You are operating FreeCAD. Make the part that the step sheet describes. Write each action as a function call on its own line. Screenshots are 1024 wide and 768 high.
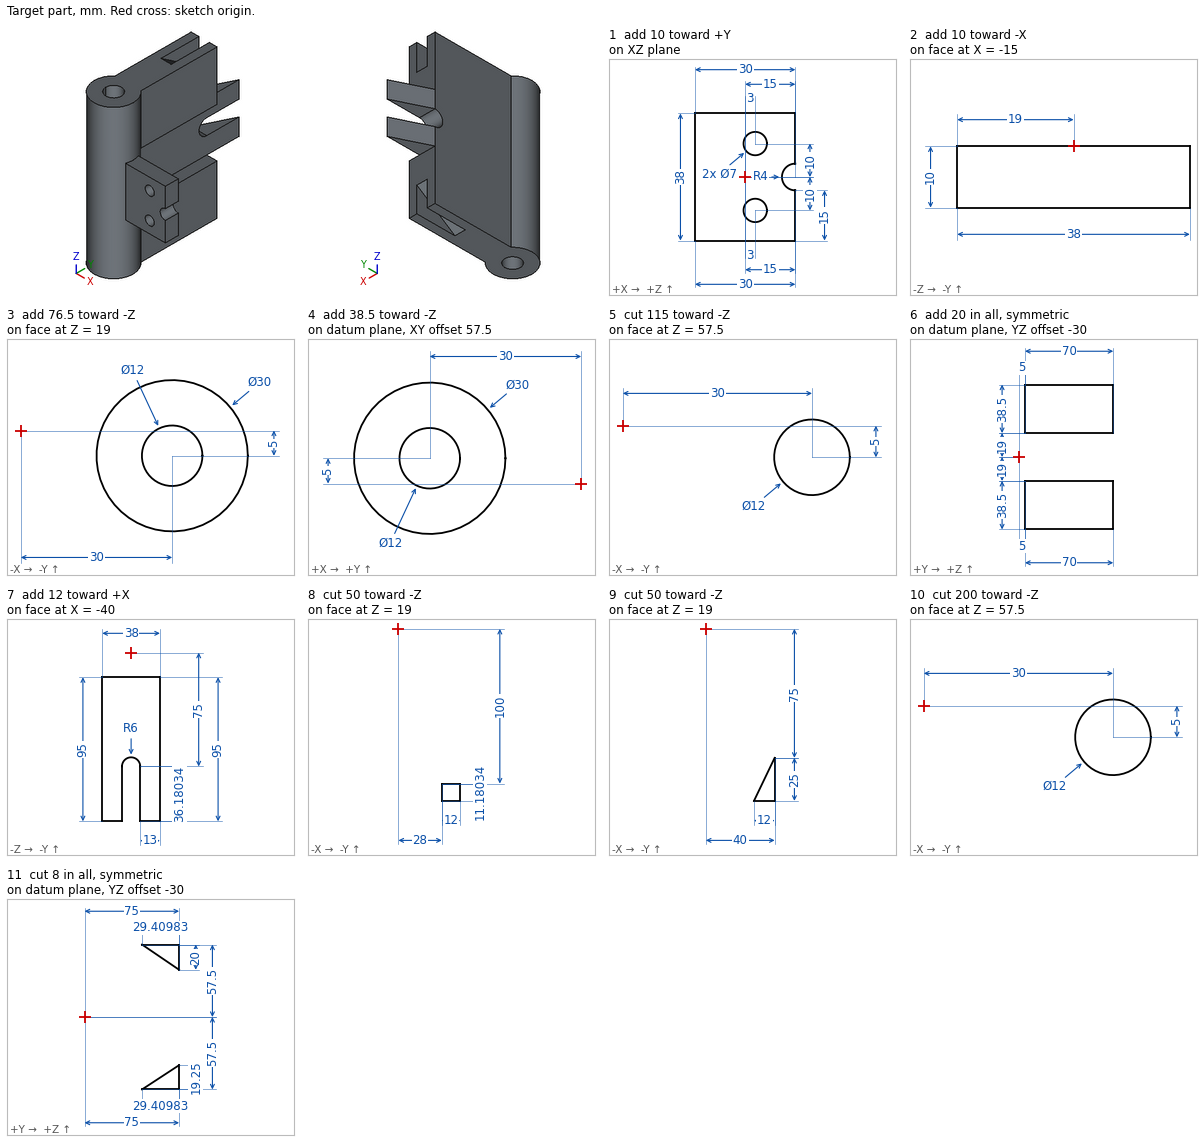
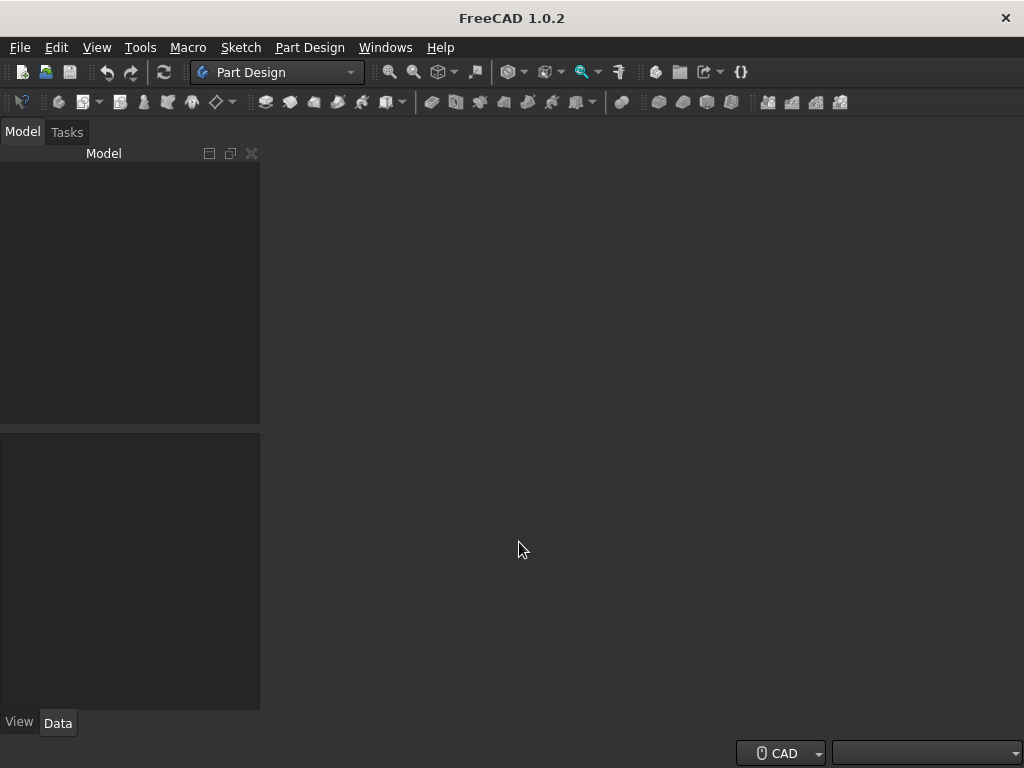
click(22, 72)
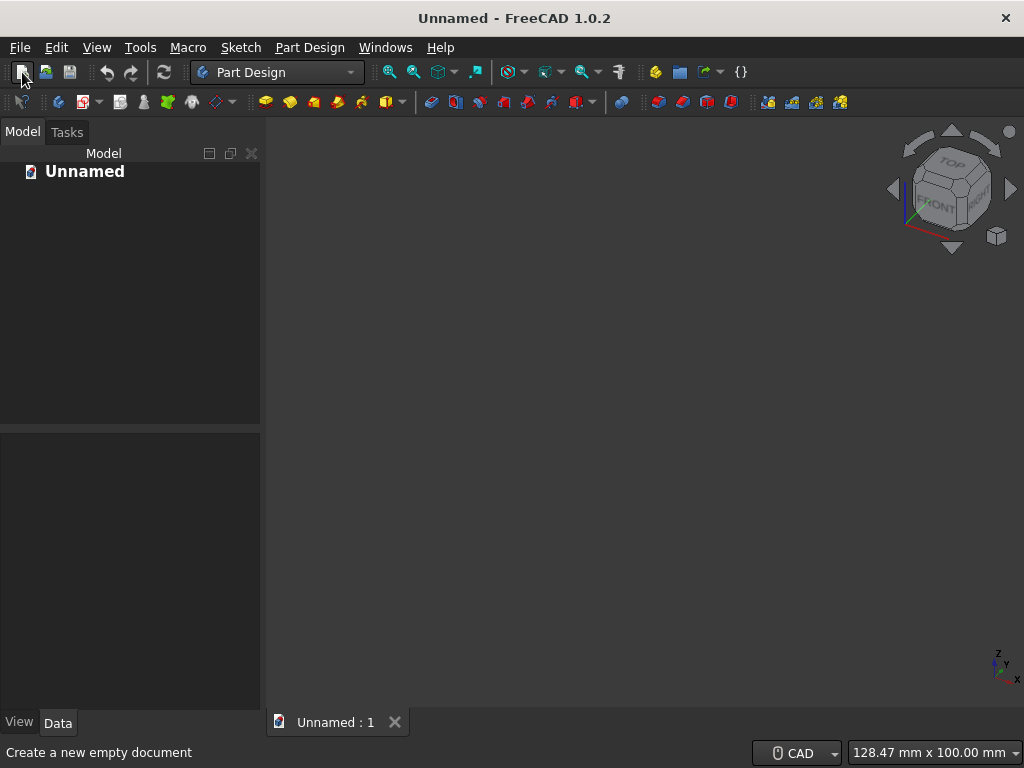
click(84, 102)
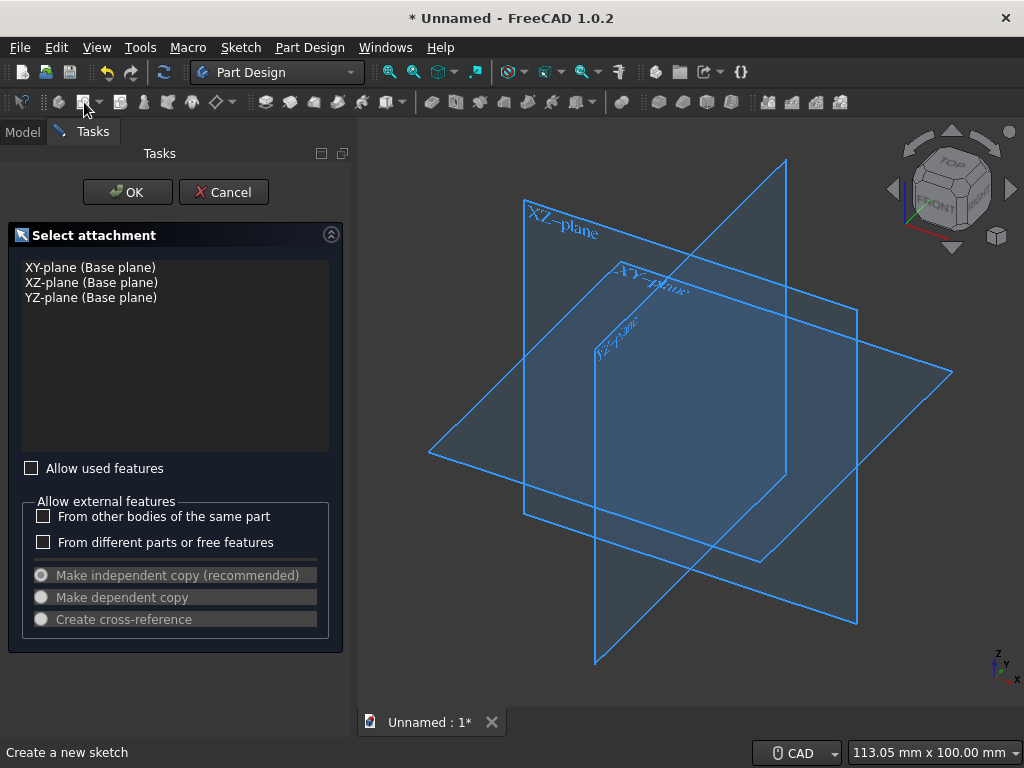
click(82, 282)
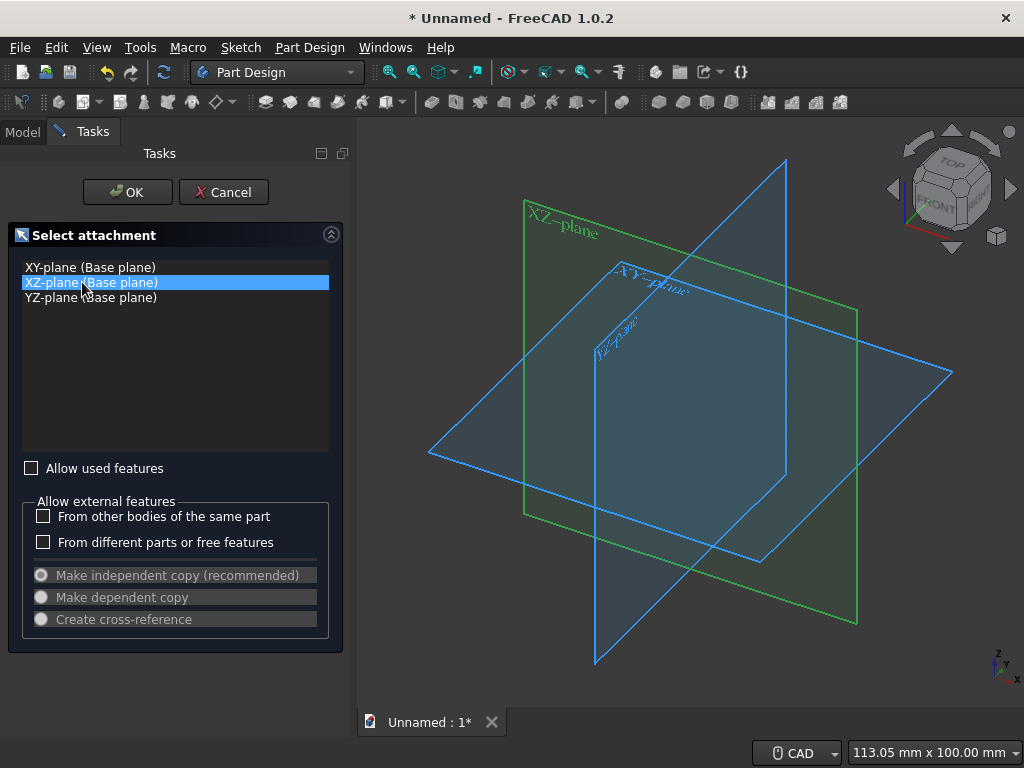
click(128, 192)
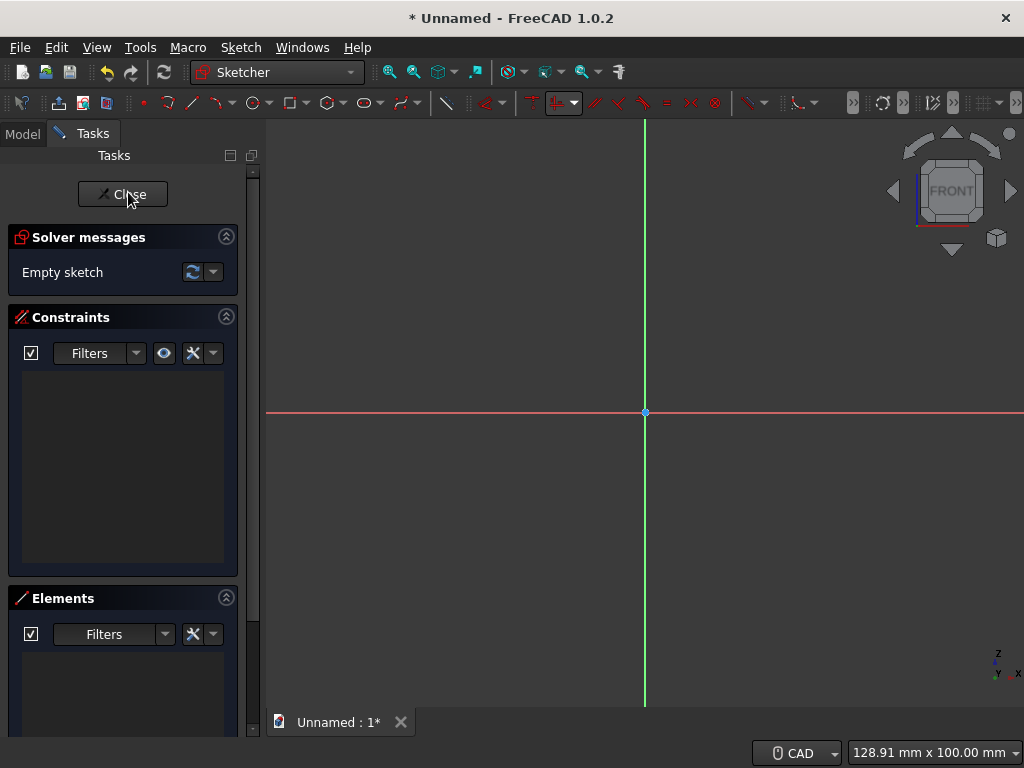
scroll(728, 413, up, 3)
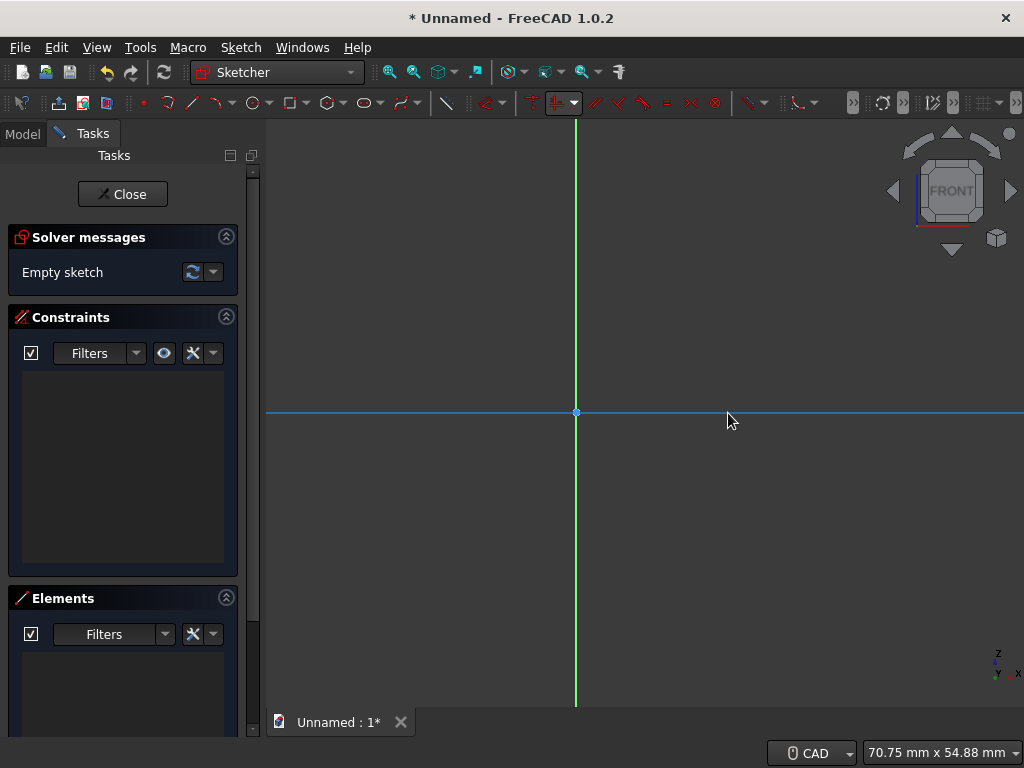
key(g)
key(m)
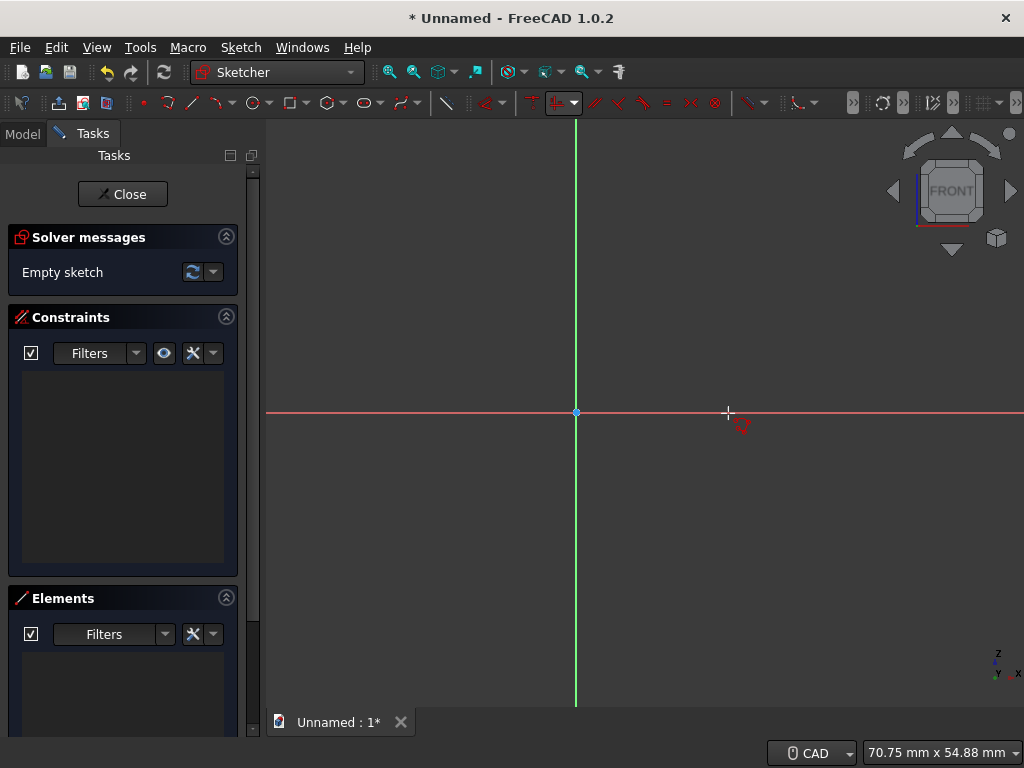
click(737, 455)
click(737, 616)
click(416, 616)
click(416, 209)
click(737, 209)
click(737, 370)
right_click(737, 370)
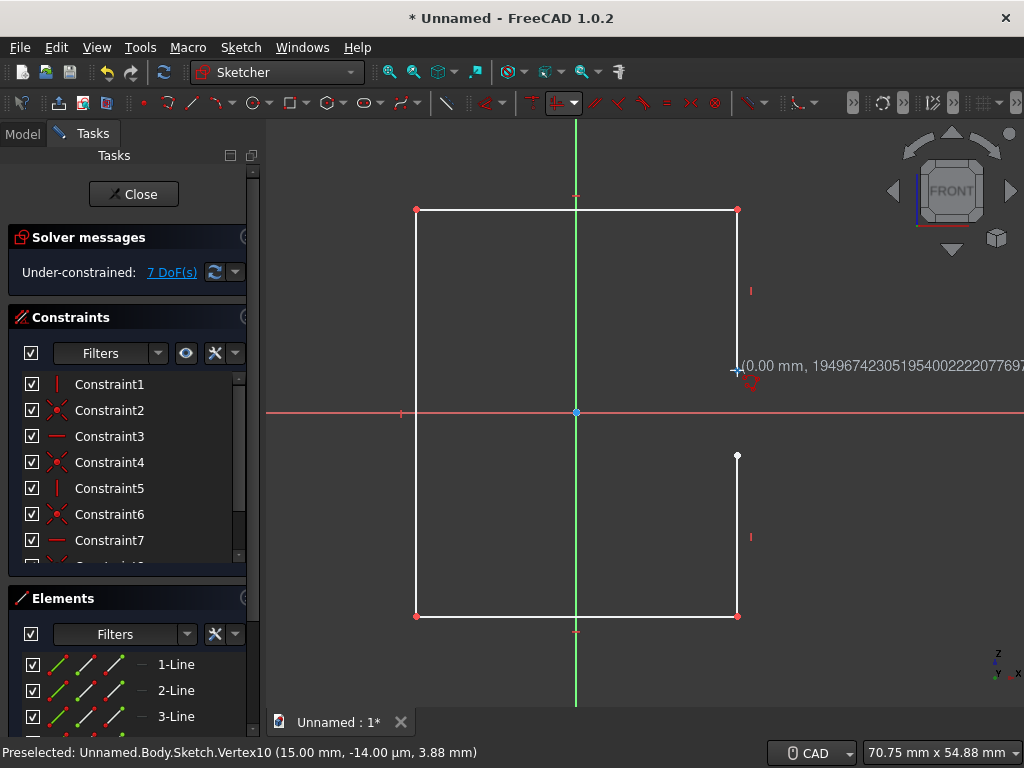
key(g)
key(3)
key(a)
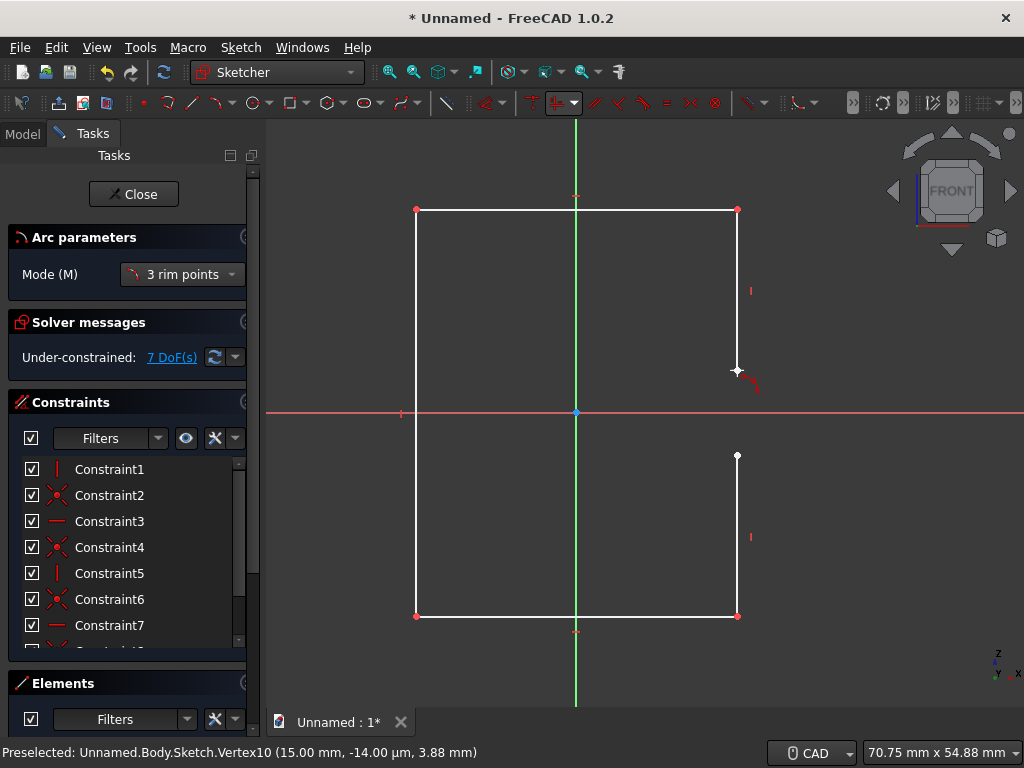
click(737, 371)
click(737, 456)
click(702, 387)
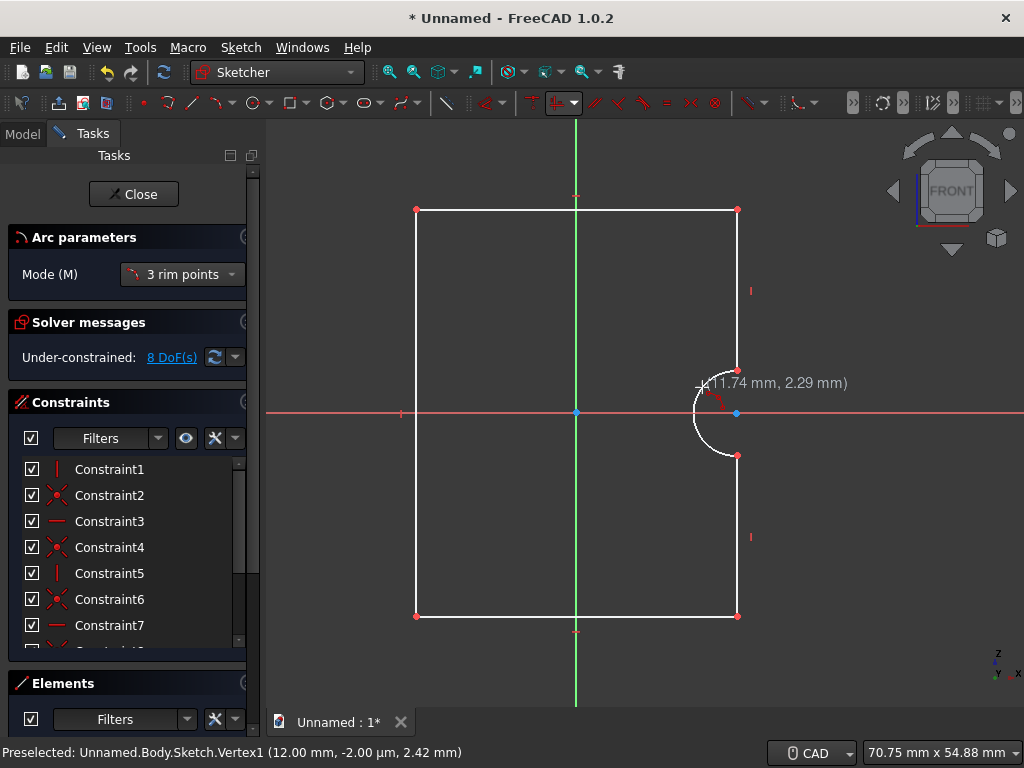
click(254, 104)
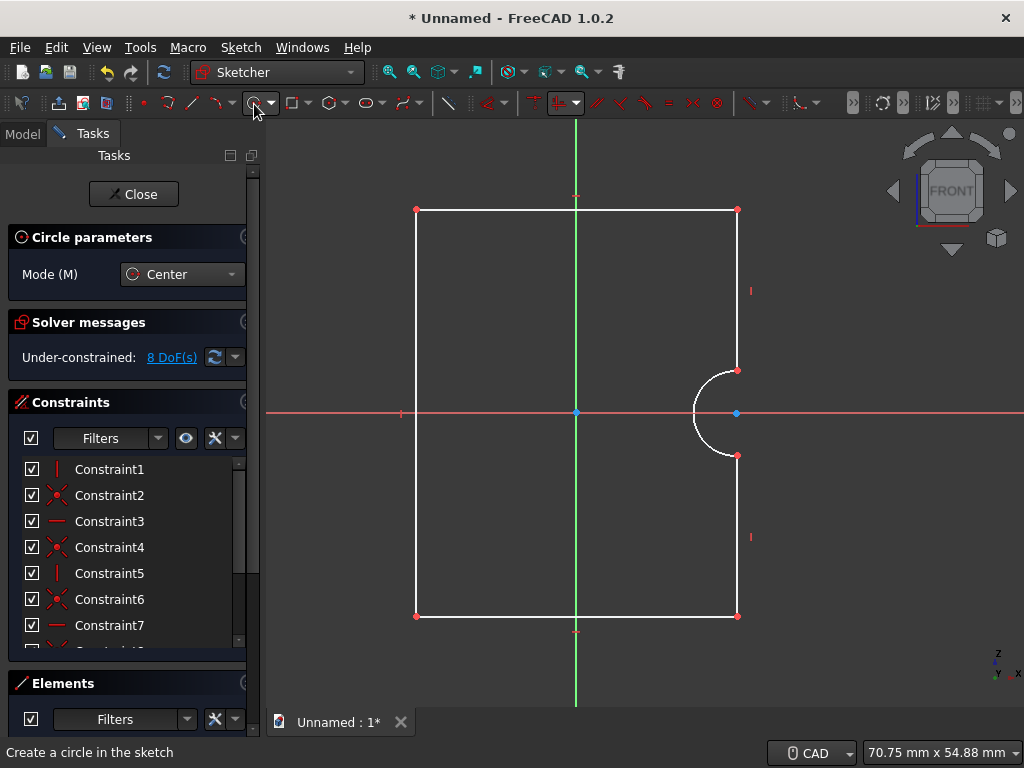
click(608, 305)
click(635, 279)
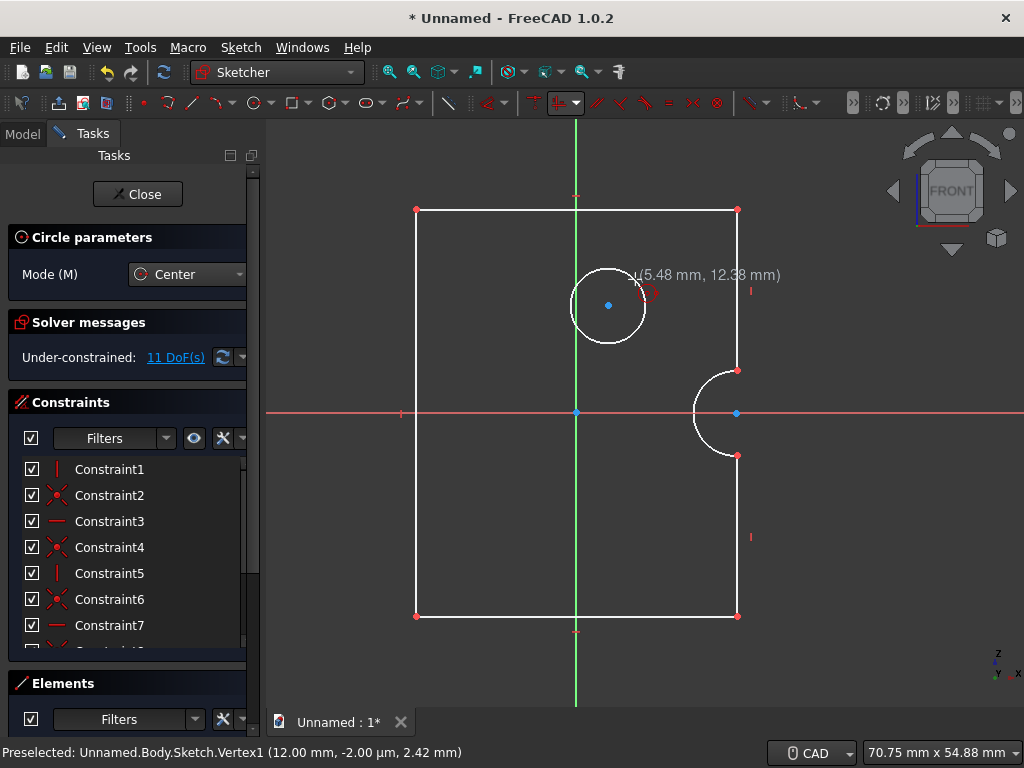
click(608, 520)
click(635, 493)
key(Escape)